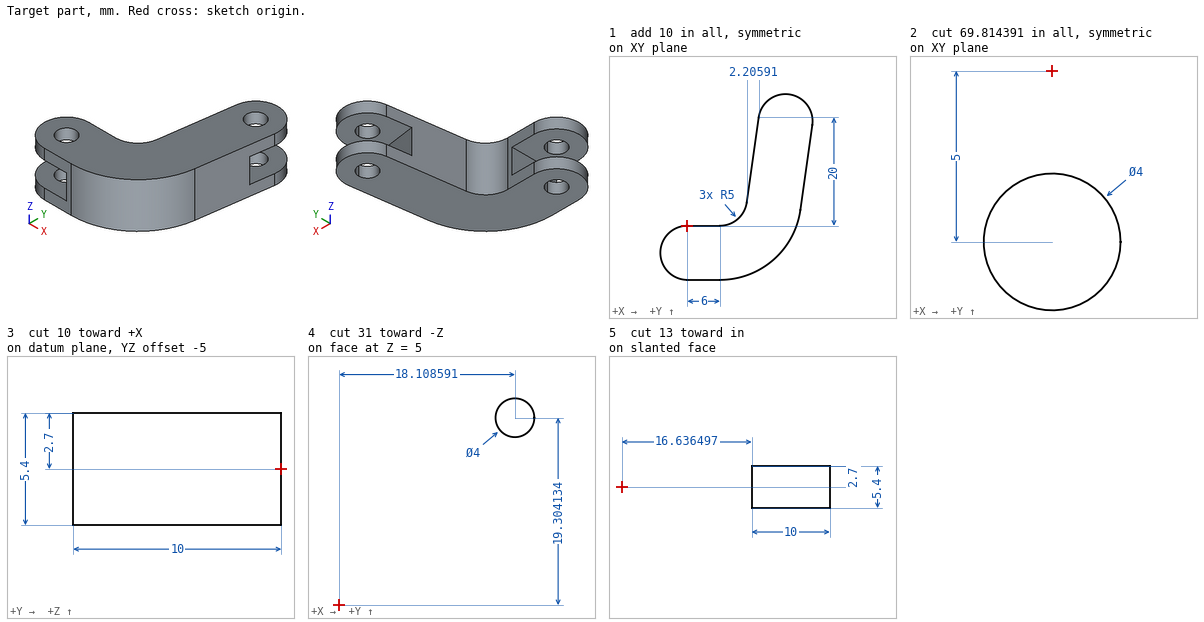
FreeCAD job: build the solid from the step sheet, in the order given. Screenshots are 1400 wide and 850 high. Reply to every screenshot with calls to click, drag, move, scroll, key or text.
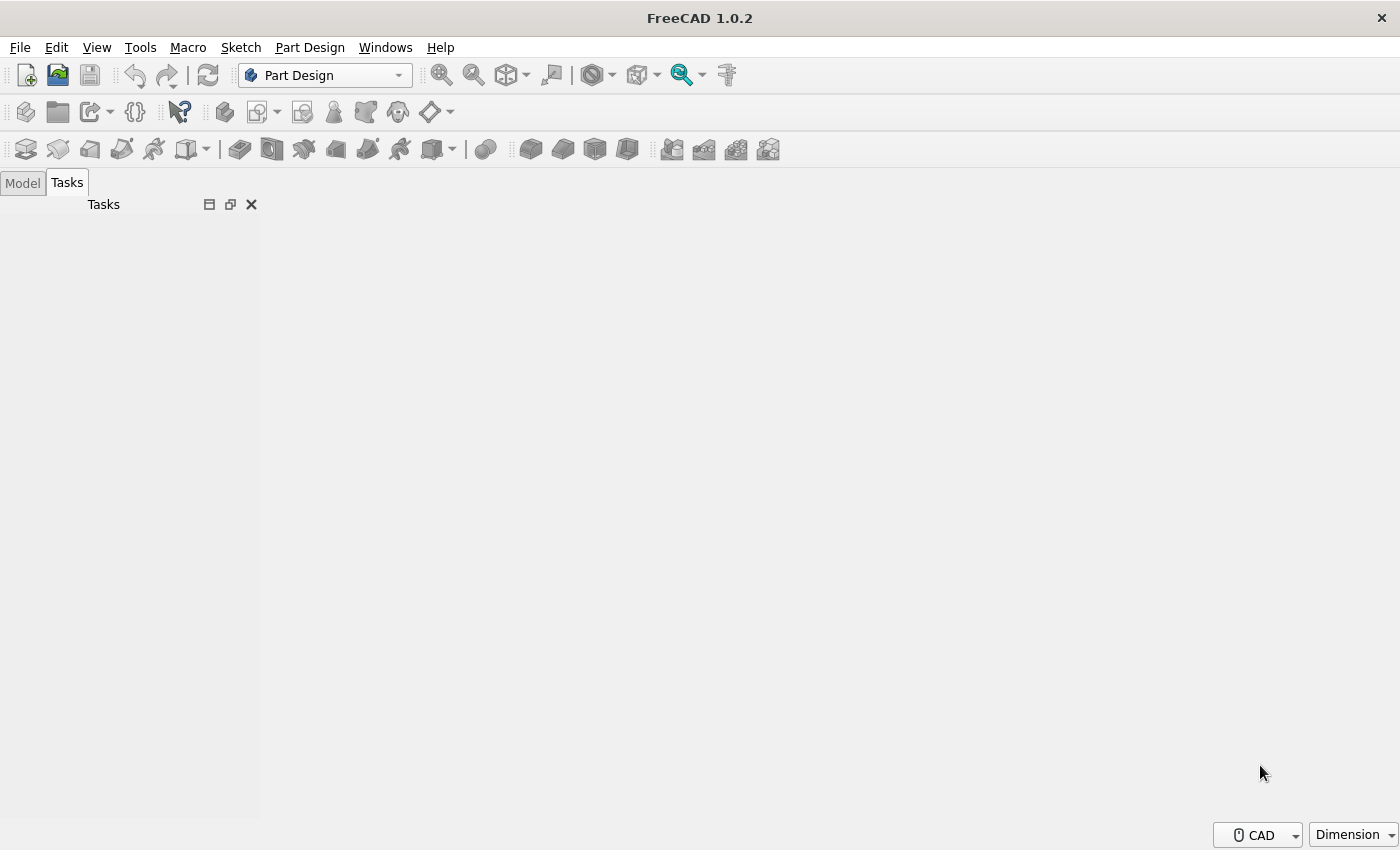
click(26, 76)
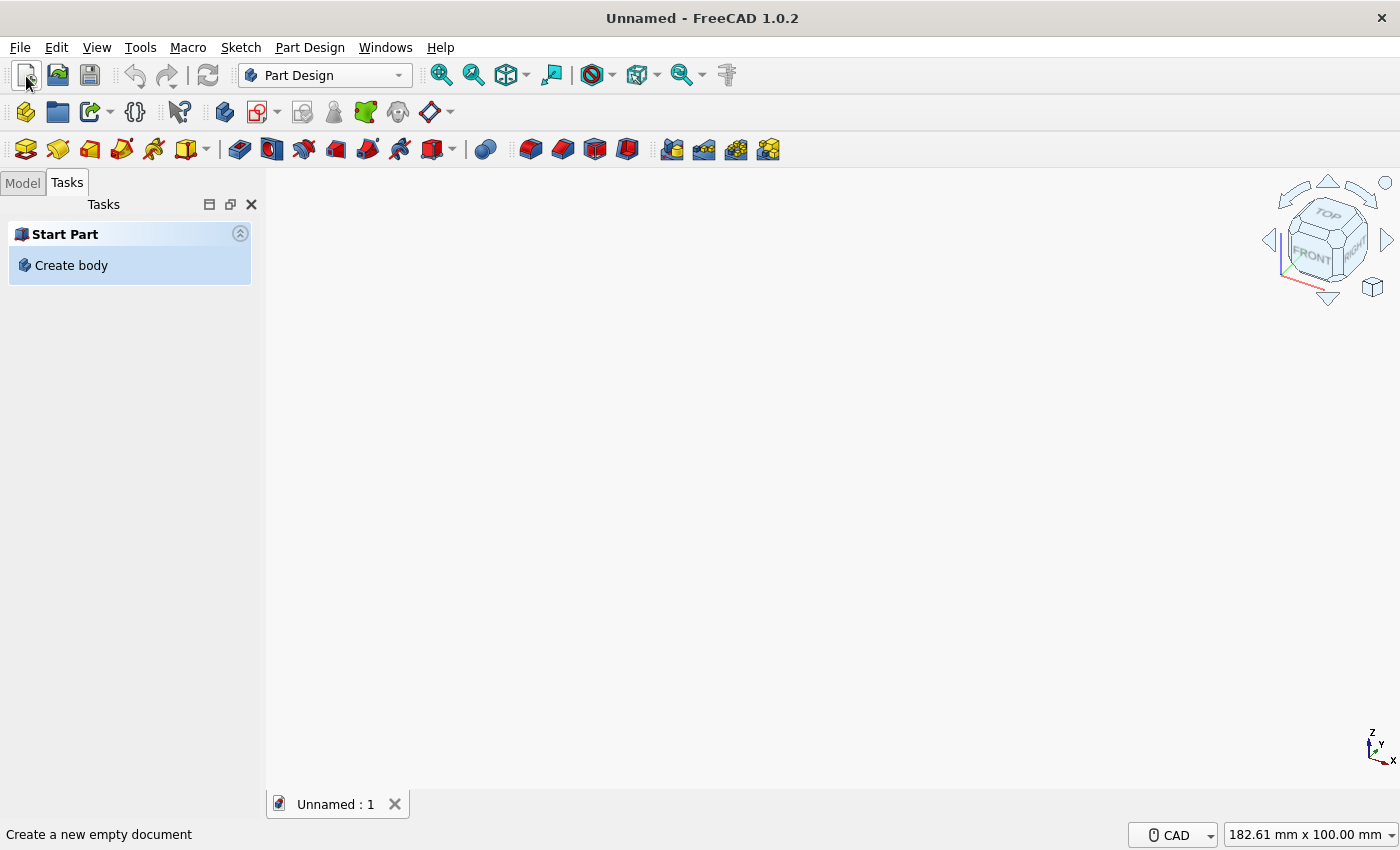
click(258, 112)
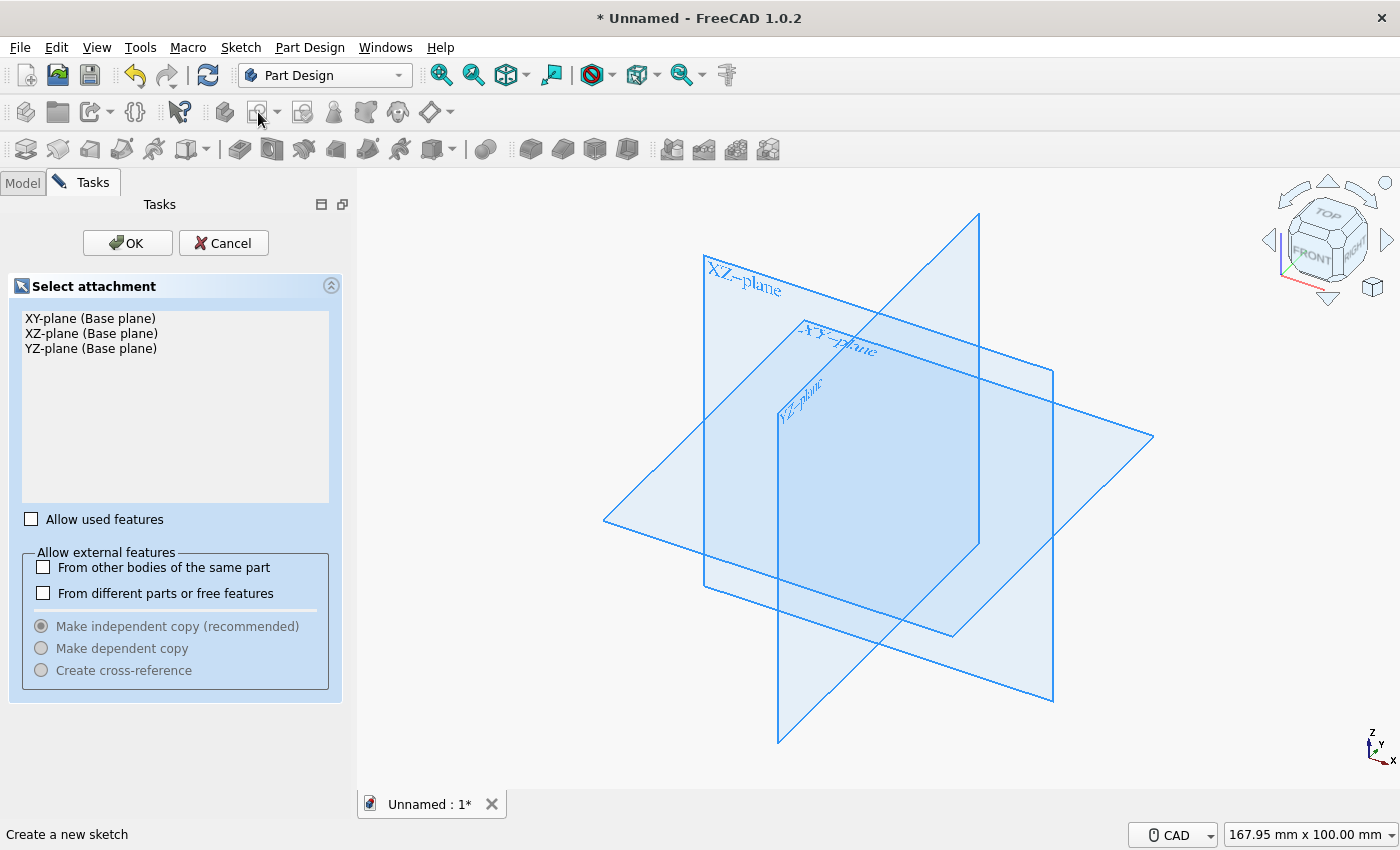
click(82, 318)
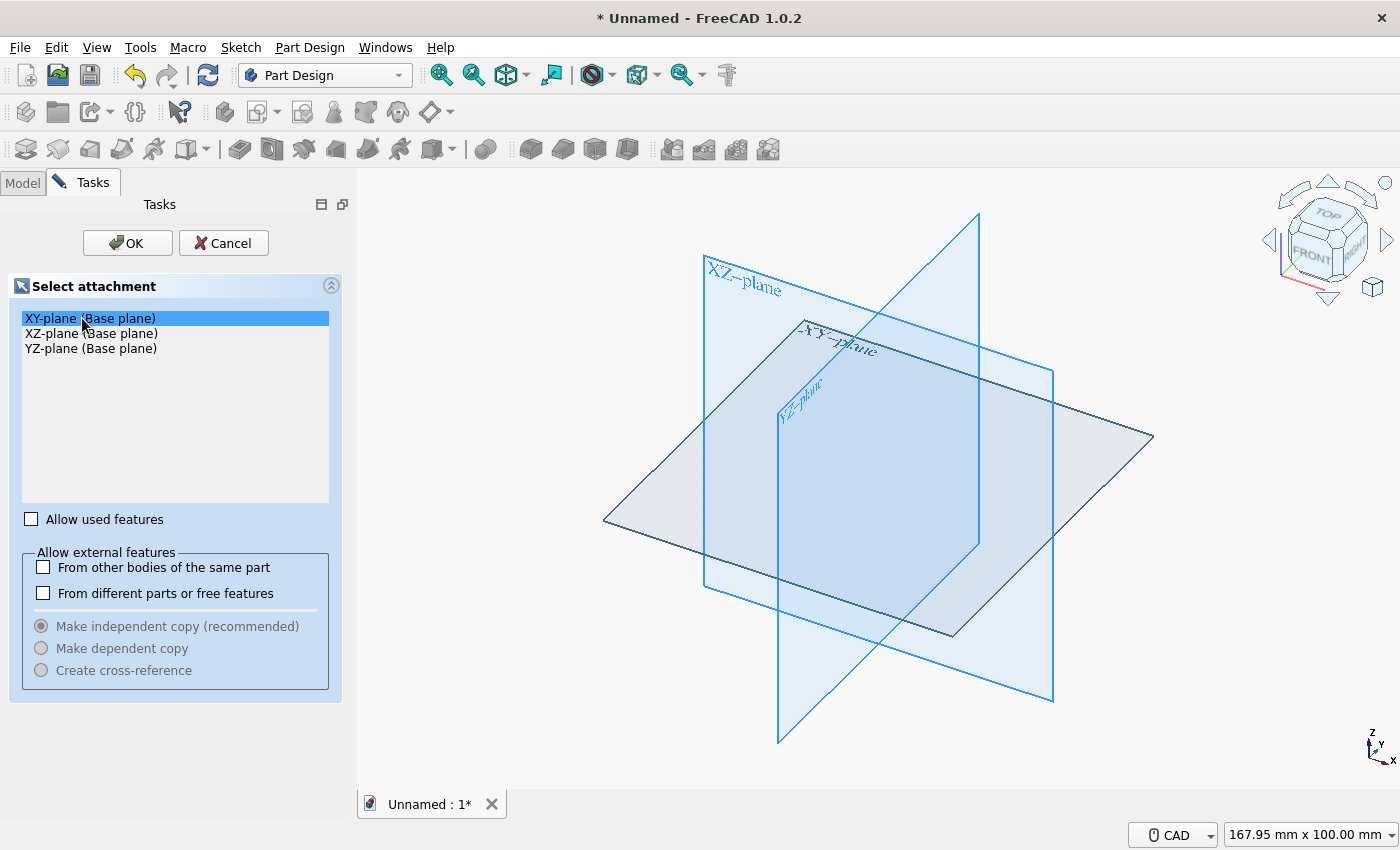
click(128, 243)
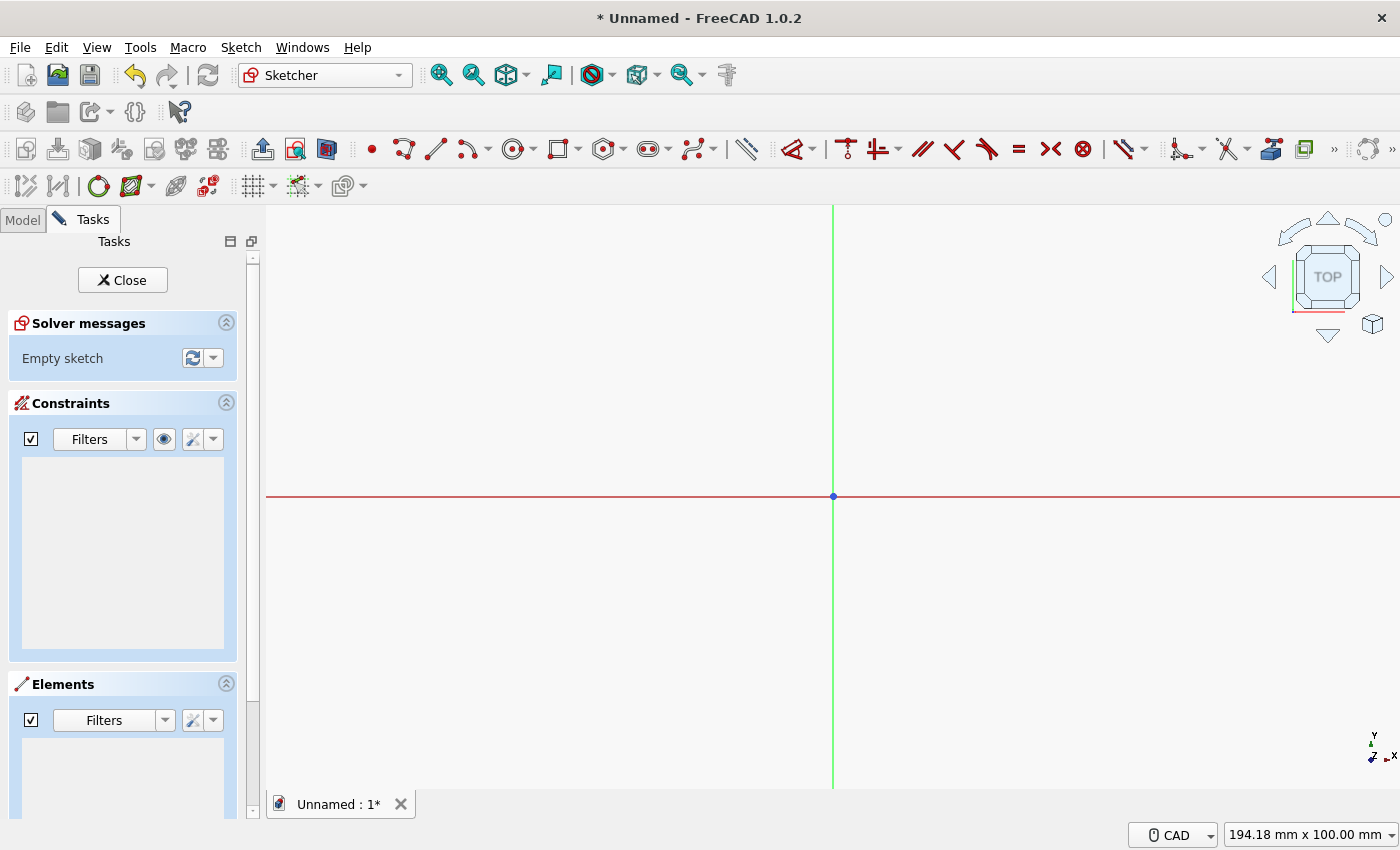
scroll(1033, 405, up, 3)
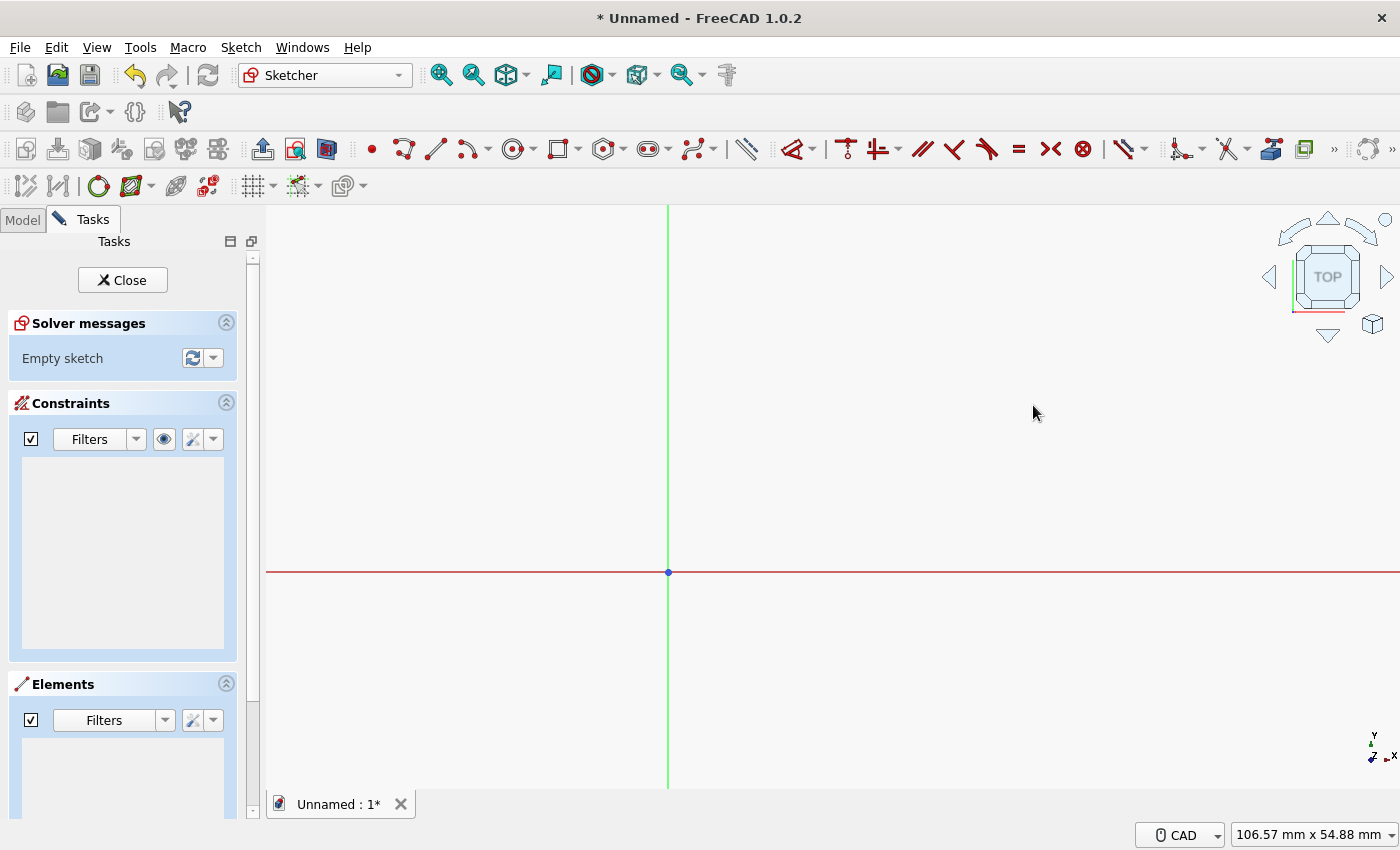
key(g)
key(l)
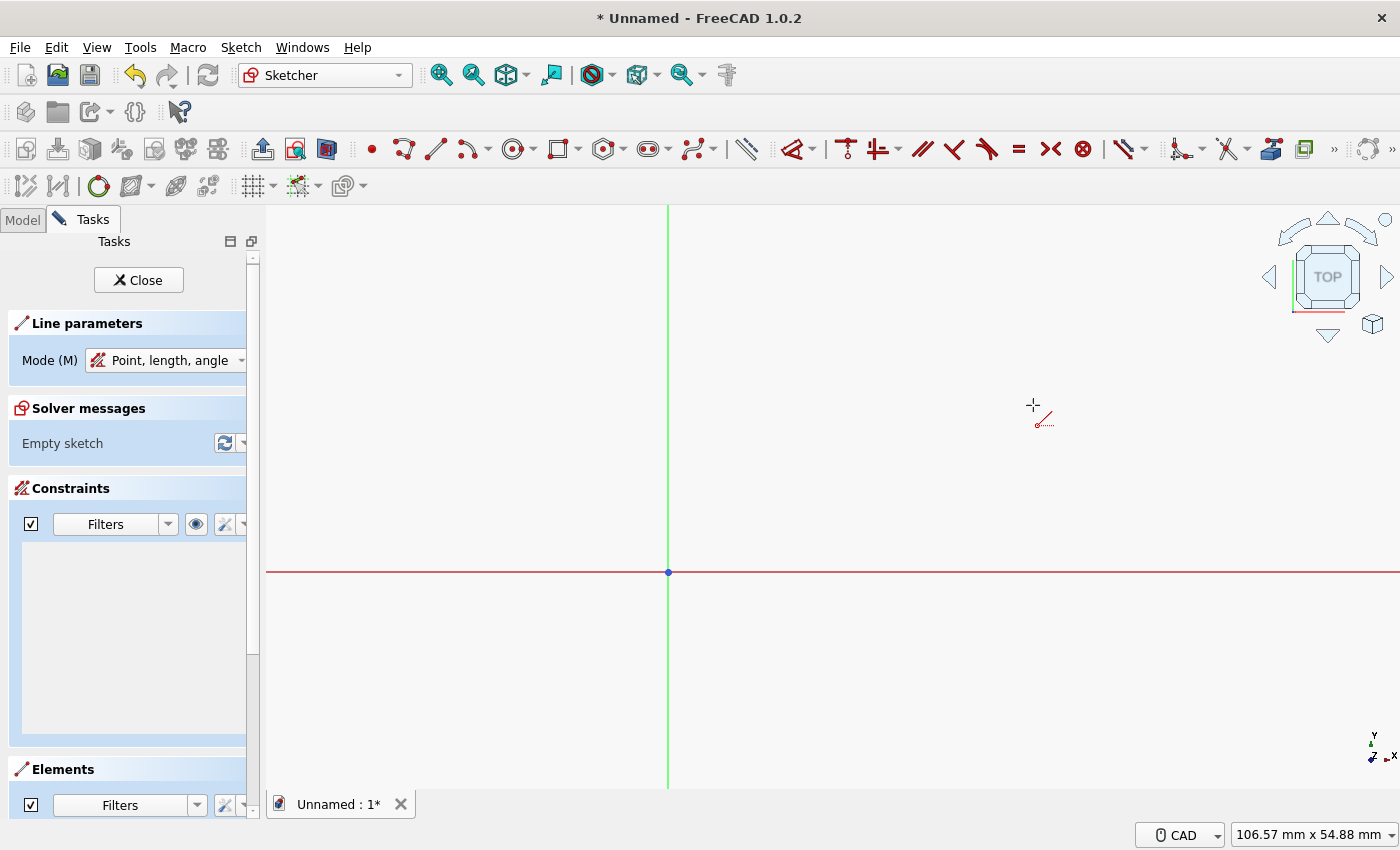
click(808, 360)
click(785, 527)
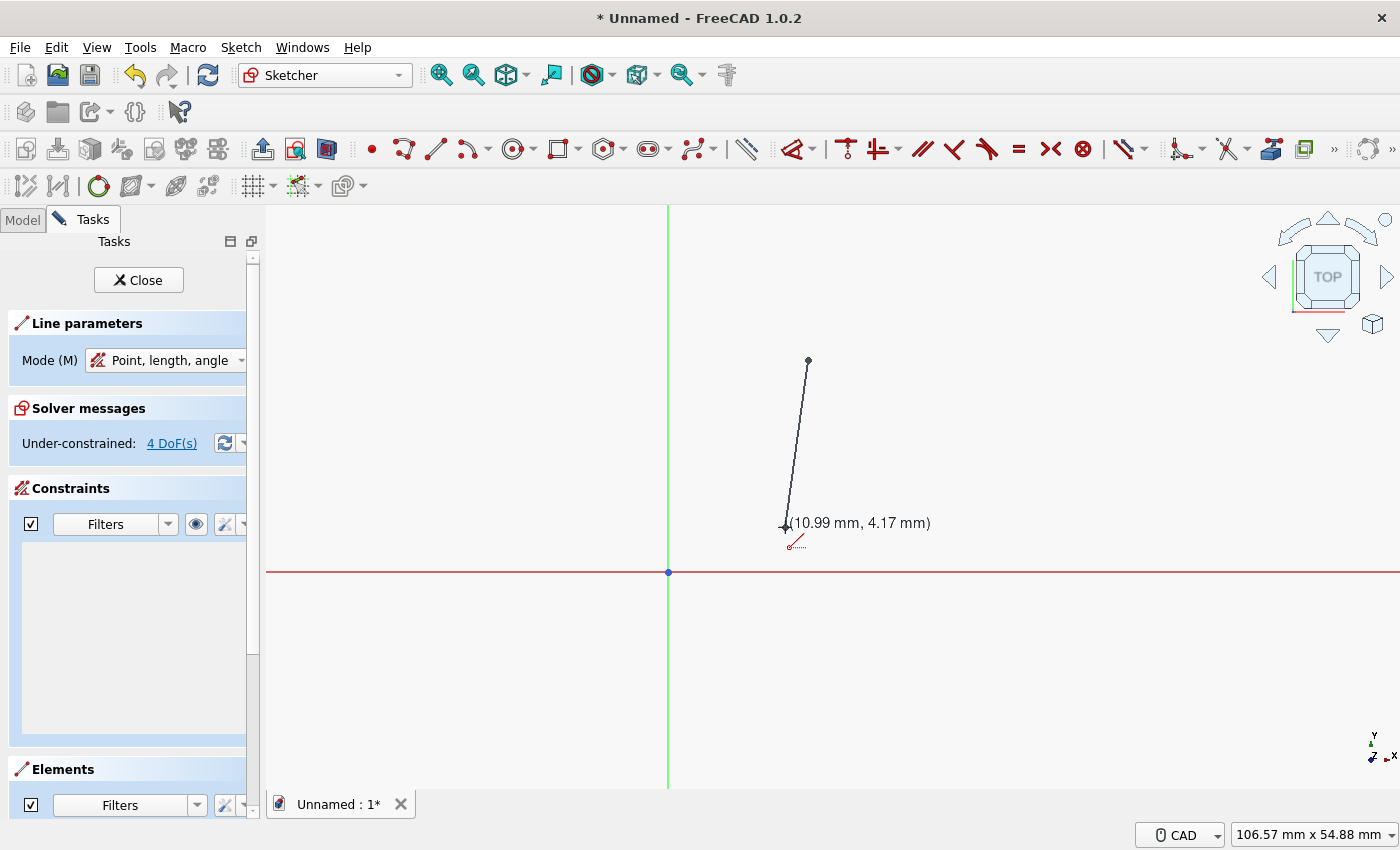
click(732, 572)
click(668, 572)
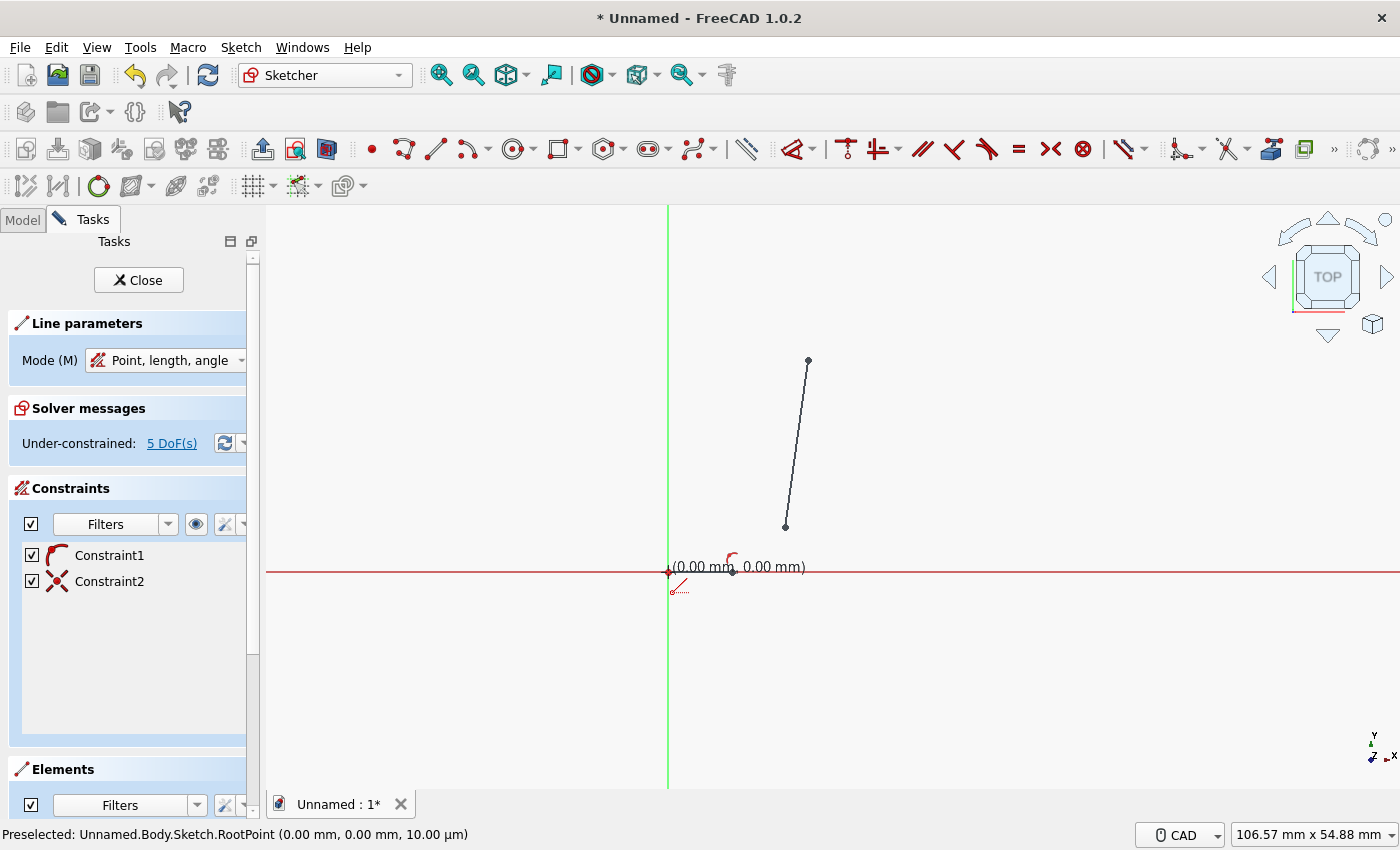
click(668, 679)
click(732, 679)